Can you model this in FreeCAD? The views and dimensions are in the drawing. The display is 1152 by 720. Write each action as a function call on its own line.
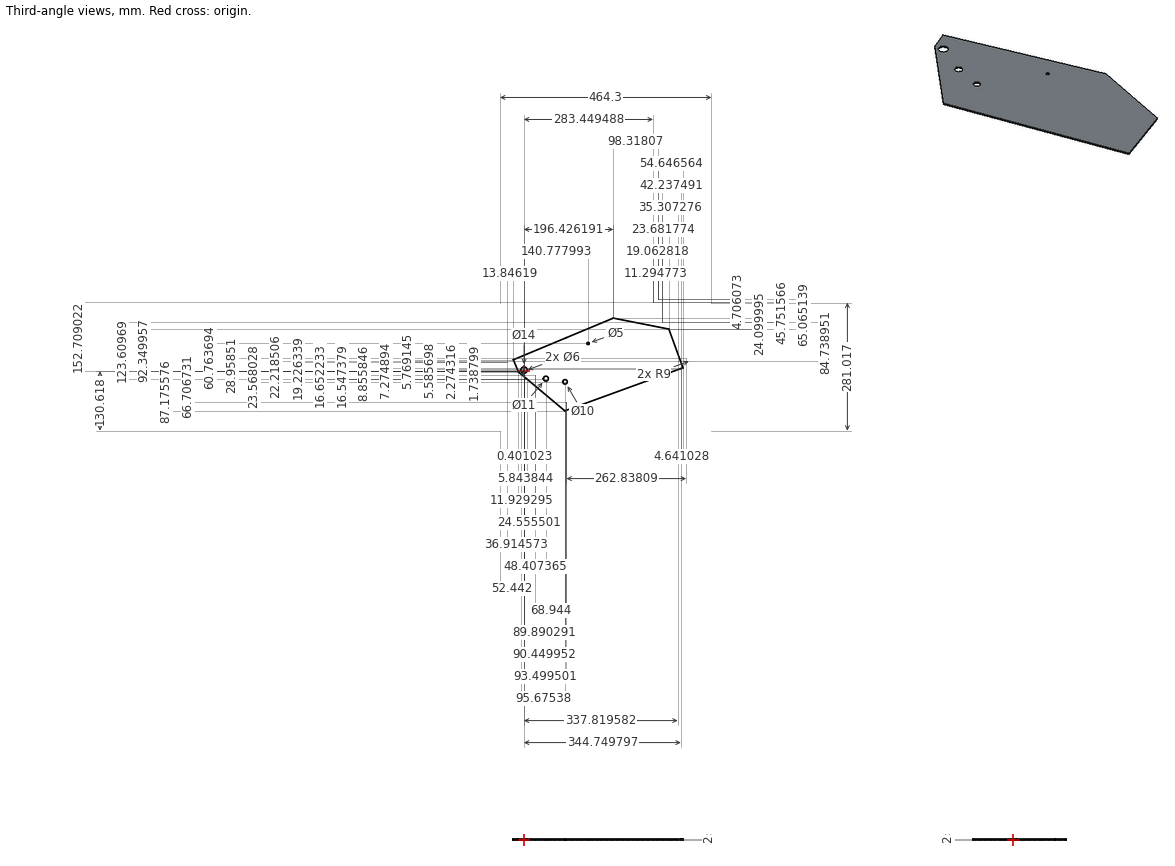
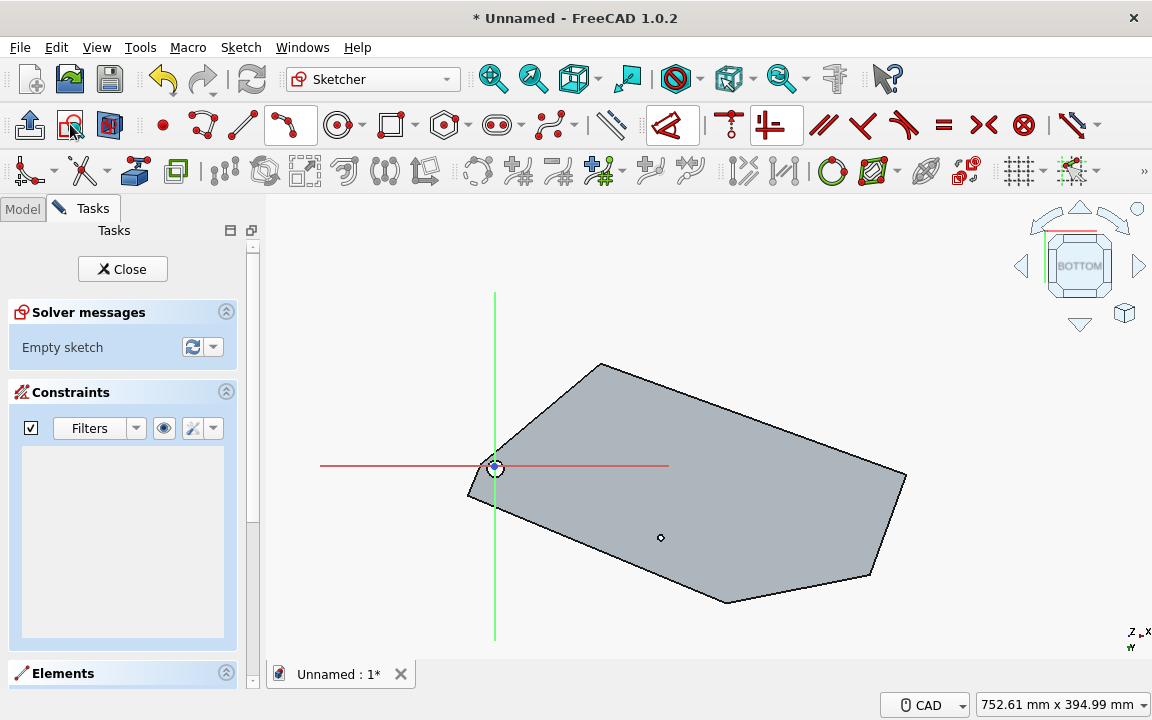
scroll(547, 448, up, 15)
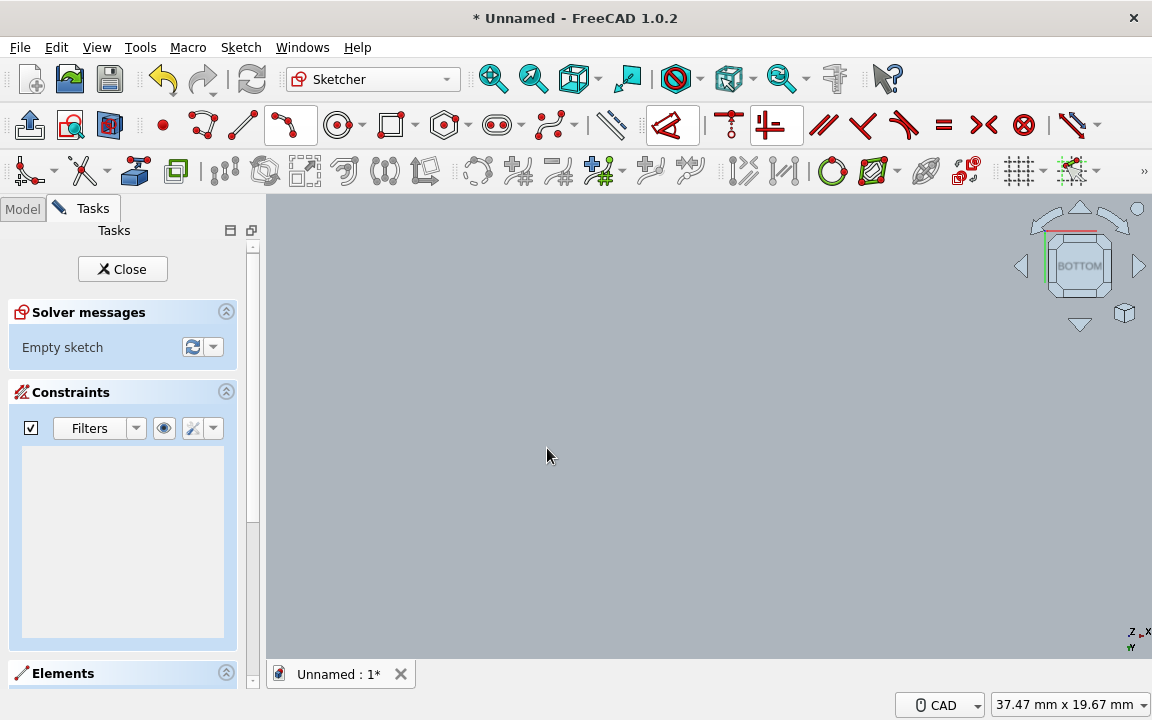
key(g)
key(c)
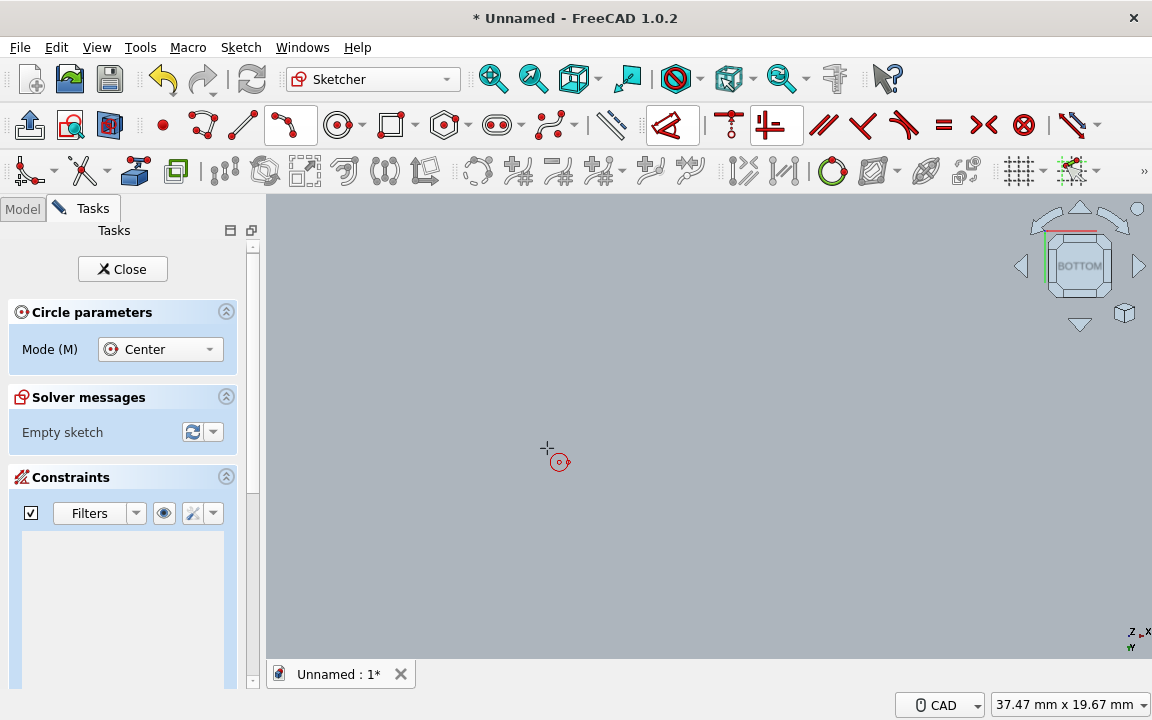
click(641, 413)
move(733, 321)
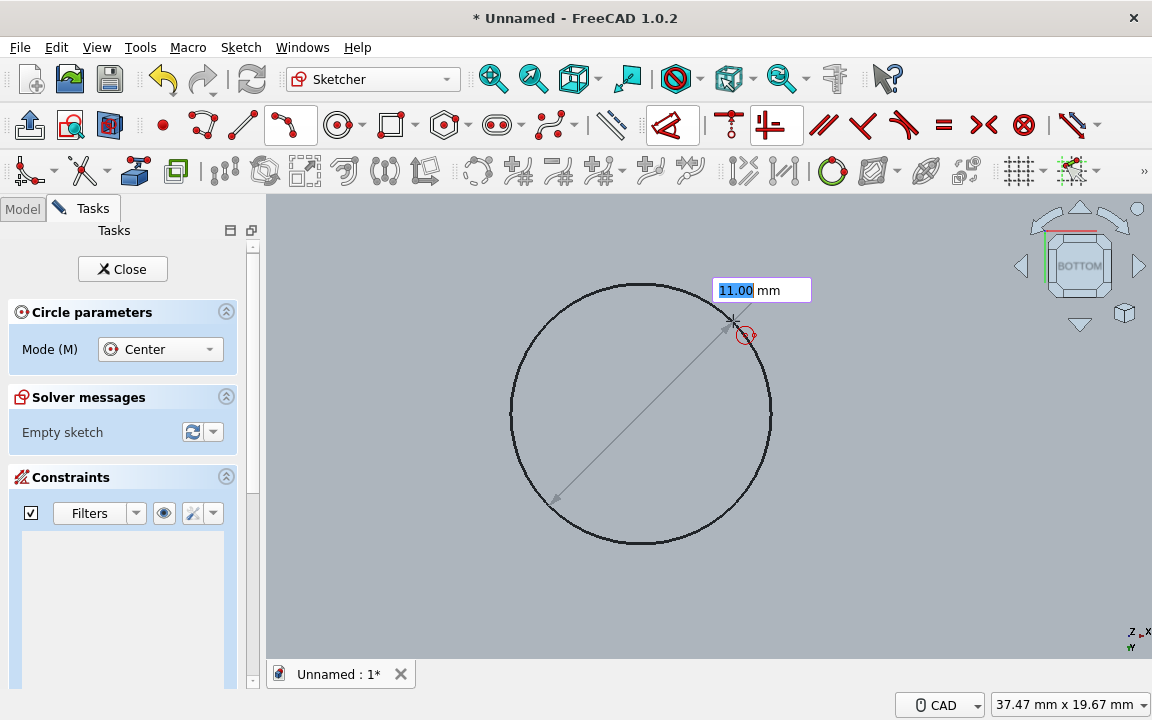
text(11)
key(Return)
key(Escape)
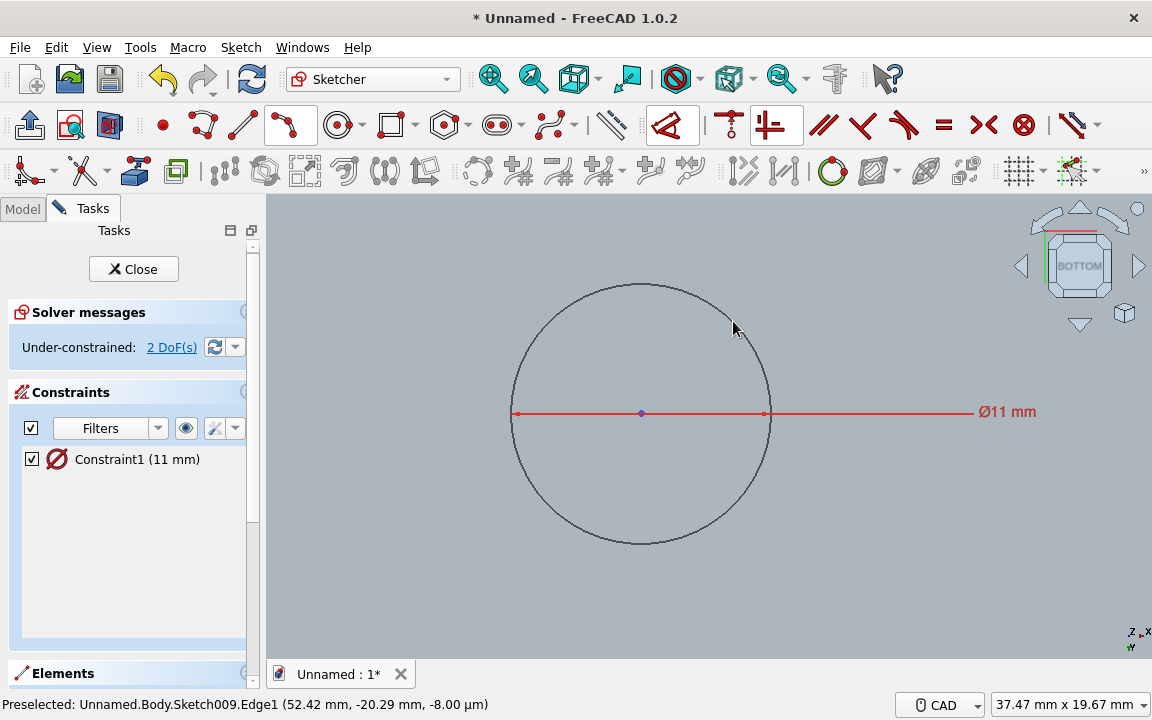
click(641, 414)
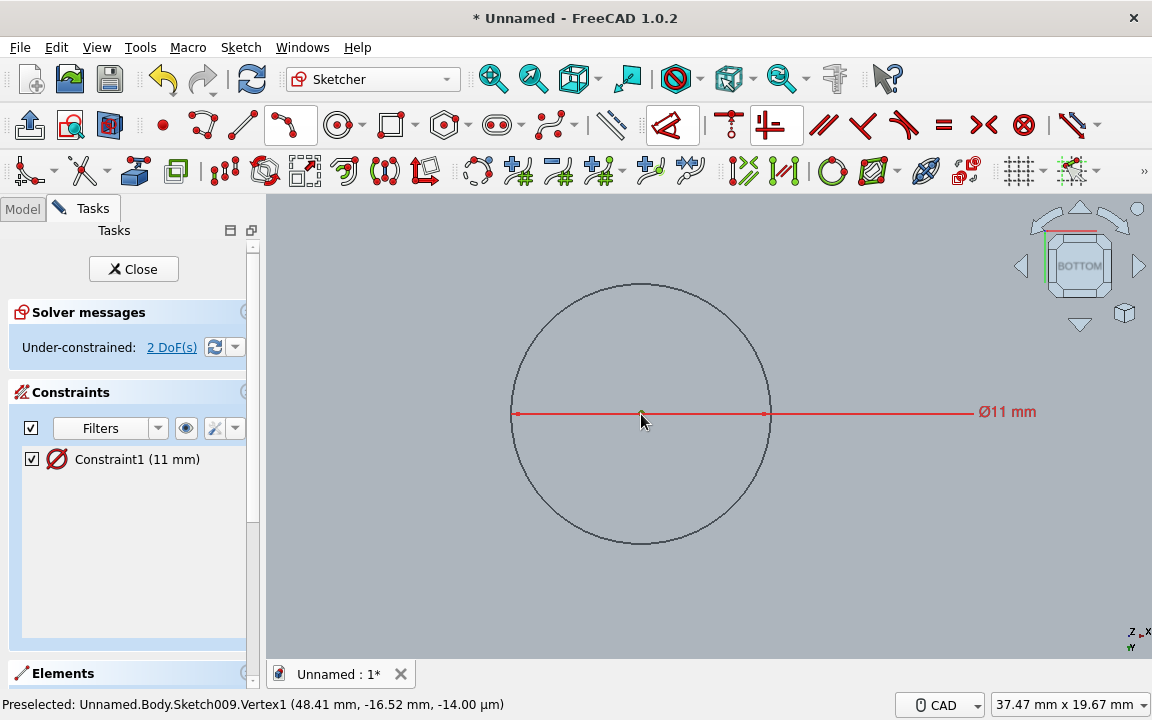
key(l)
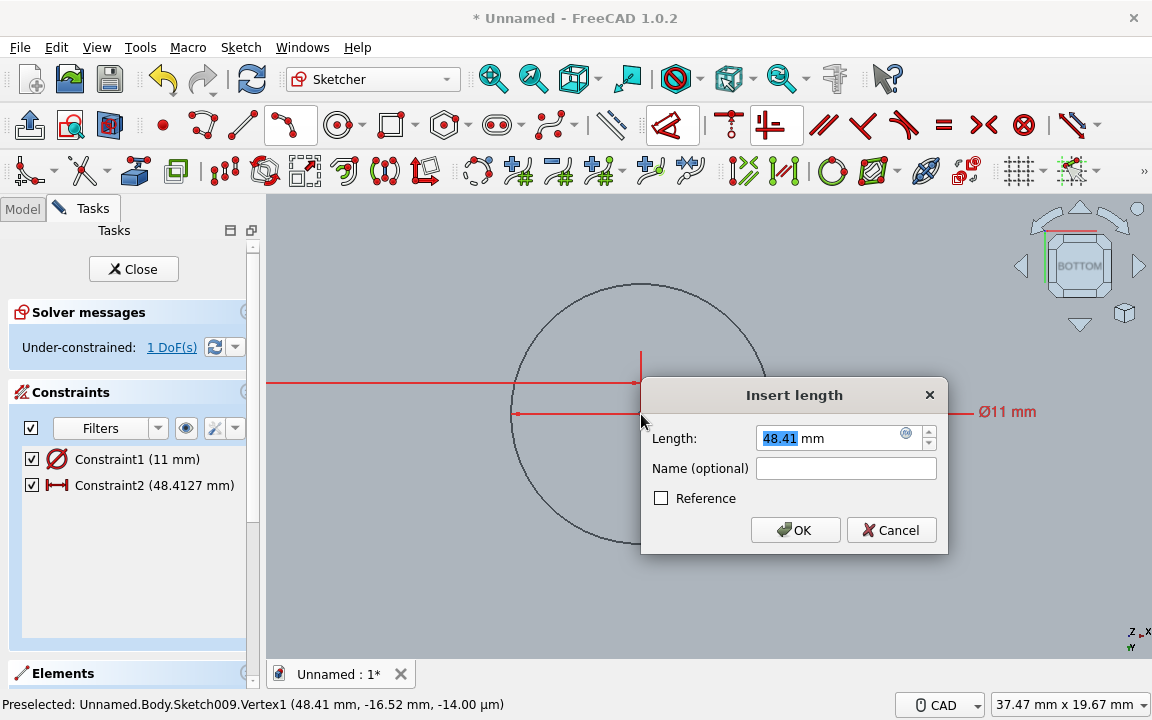
text(48.407365)
key(Return)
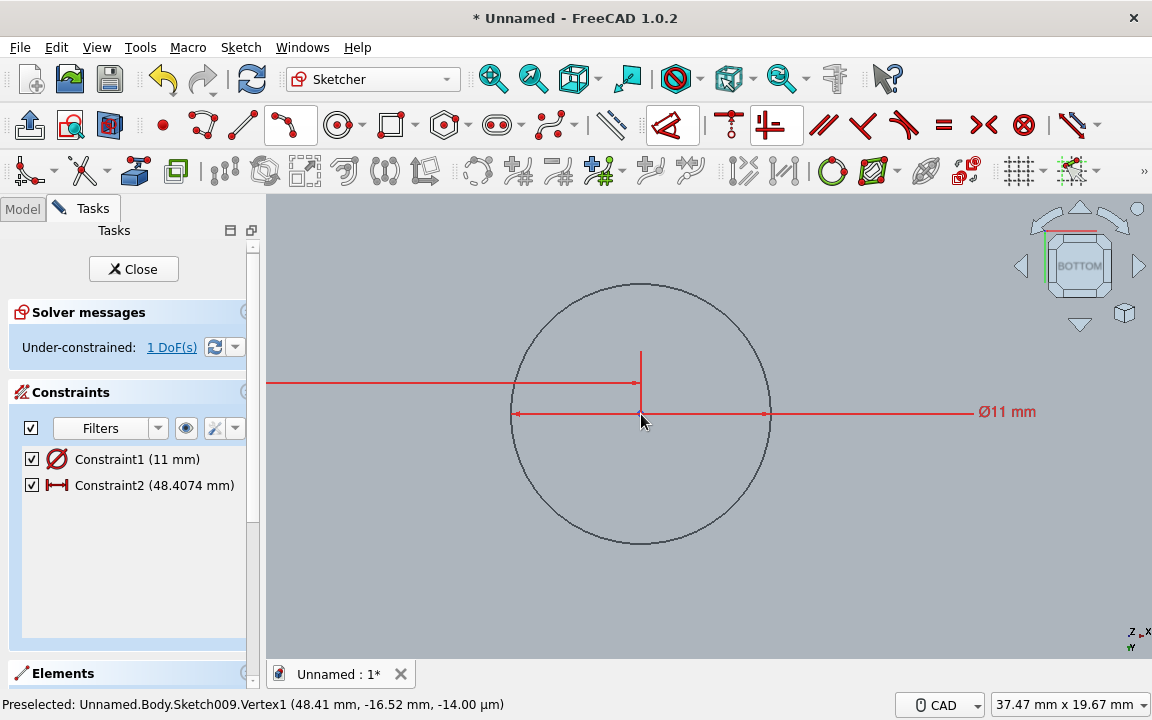
click(641, 414)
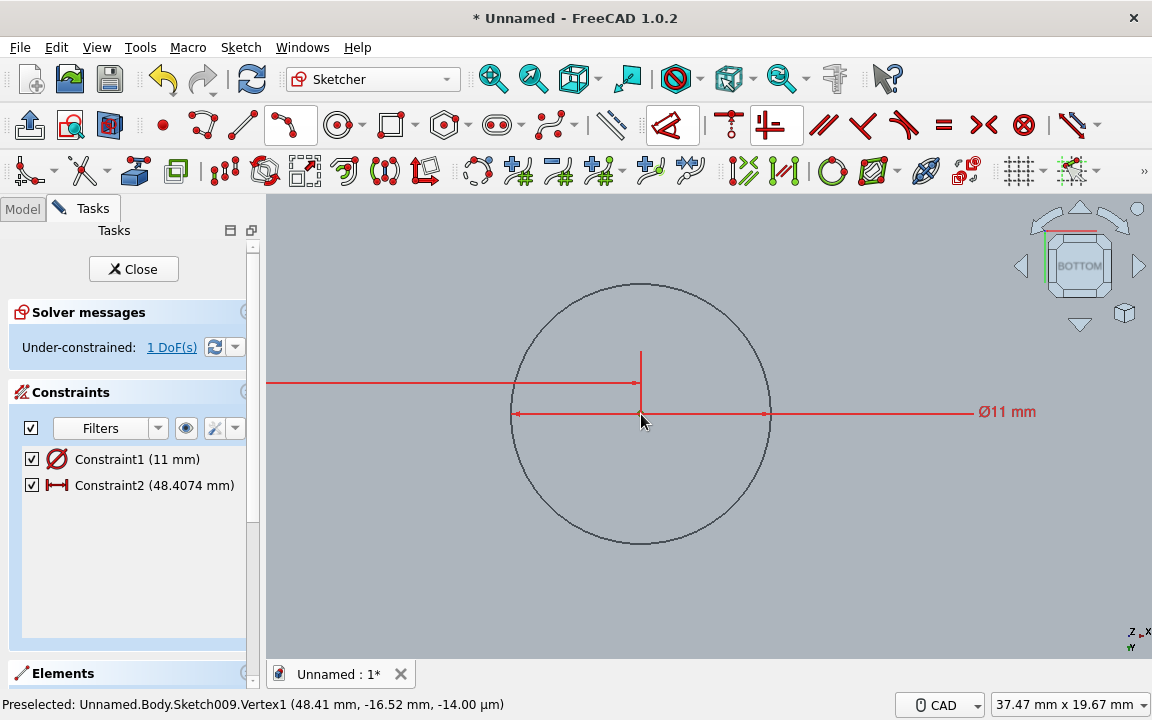
key(i)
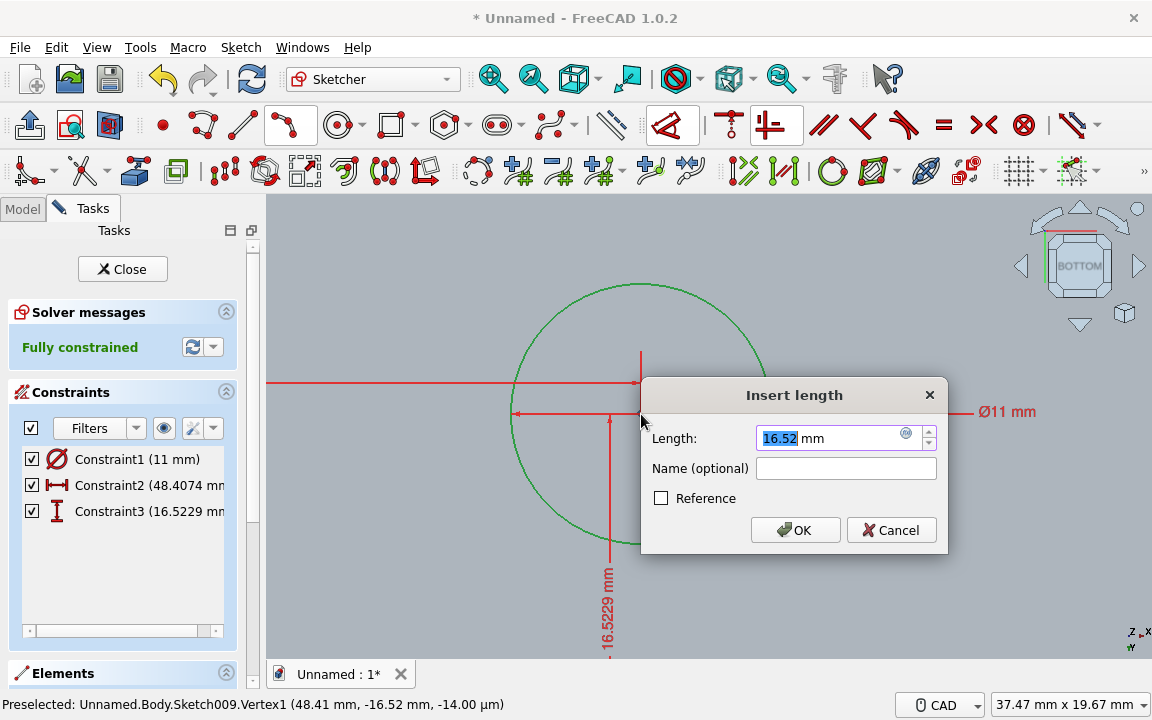
text(16.547379)
key(Return)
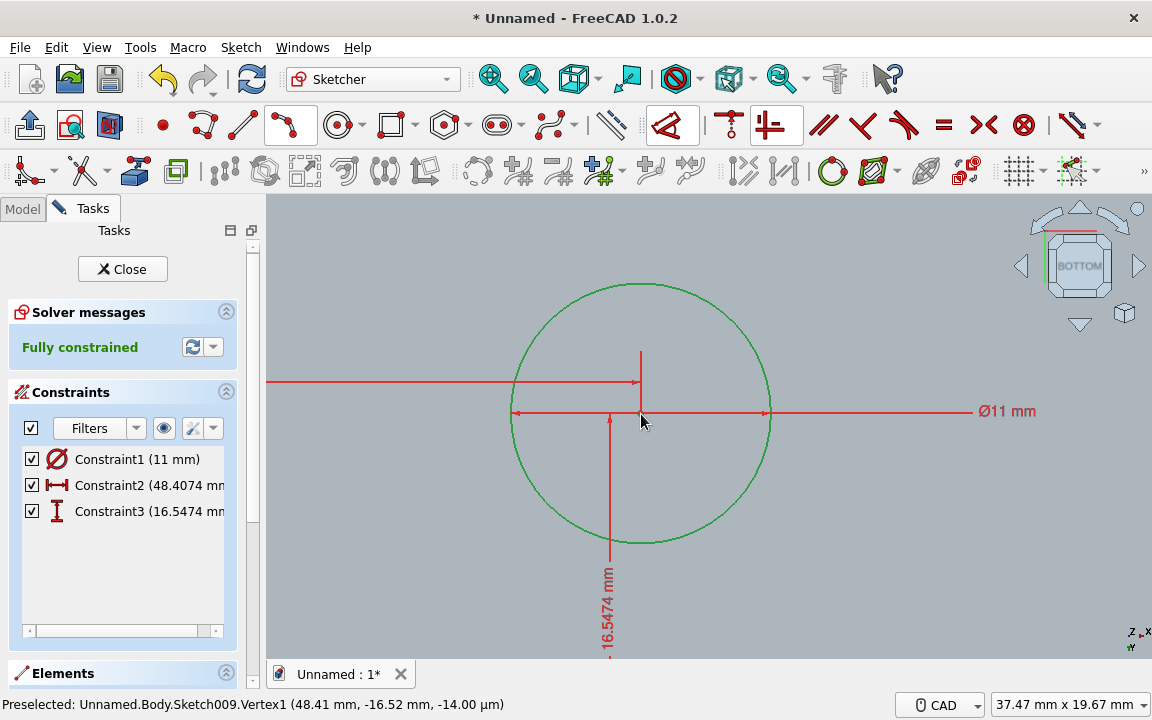
click(123, 269)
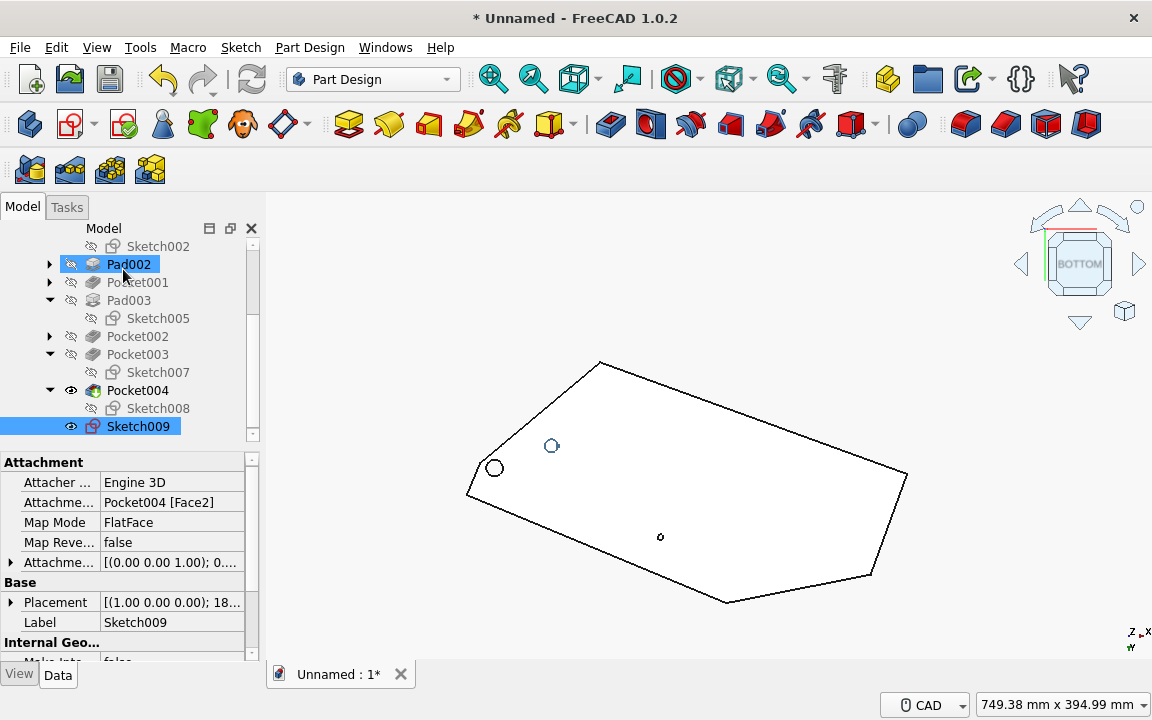
click(612, 124)